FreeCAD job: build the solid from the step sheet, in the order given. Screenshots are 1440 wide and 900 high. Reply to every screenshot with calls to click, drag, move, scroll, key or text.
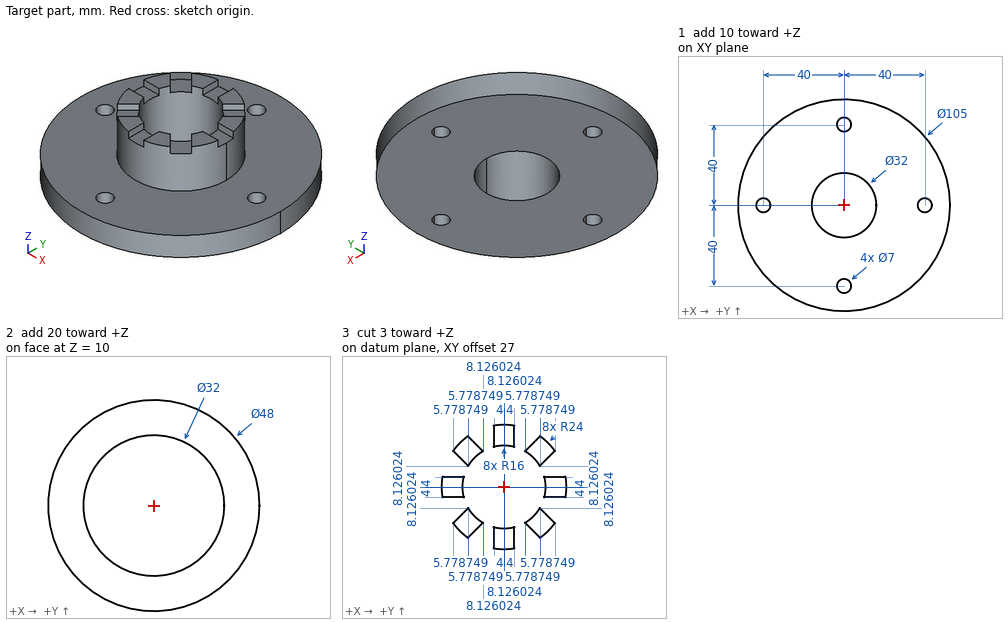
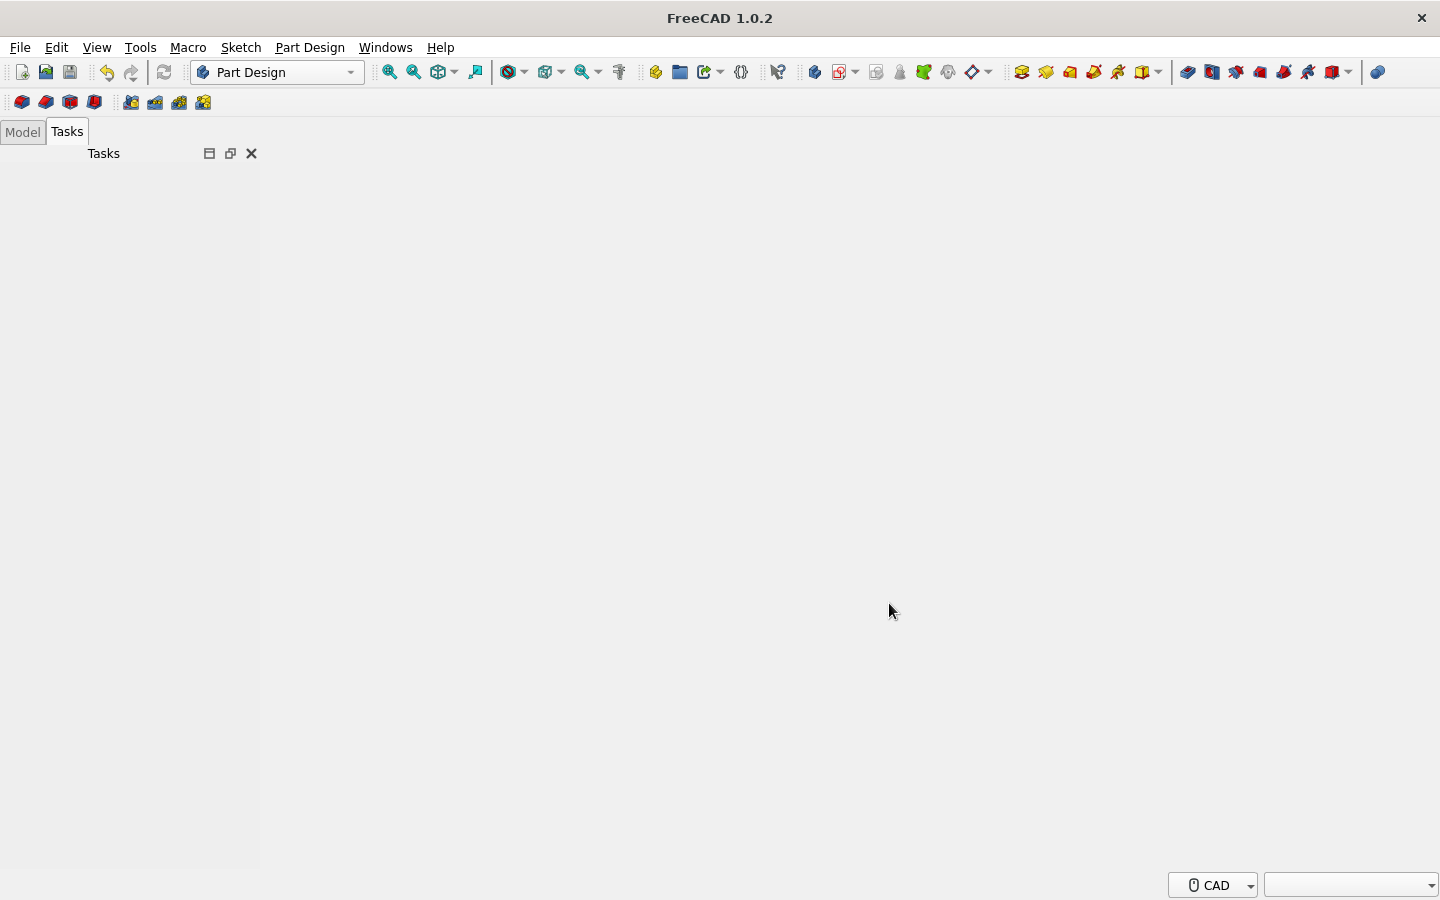
click(22, 72)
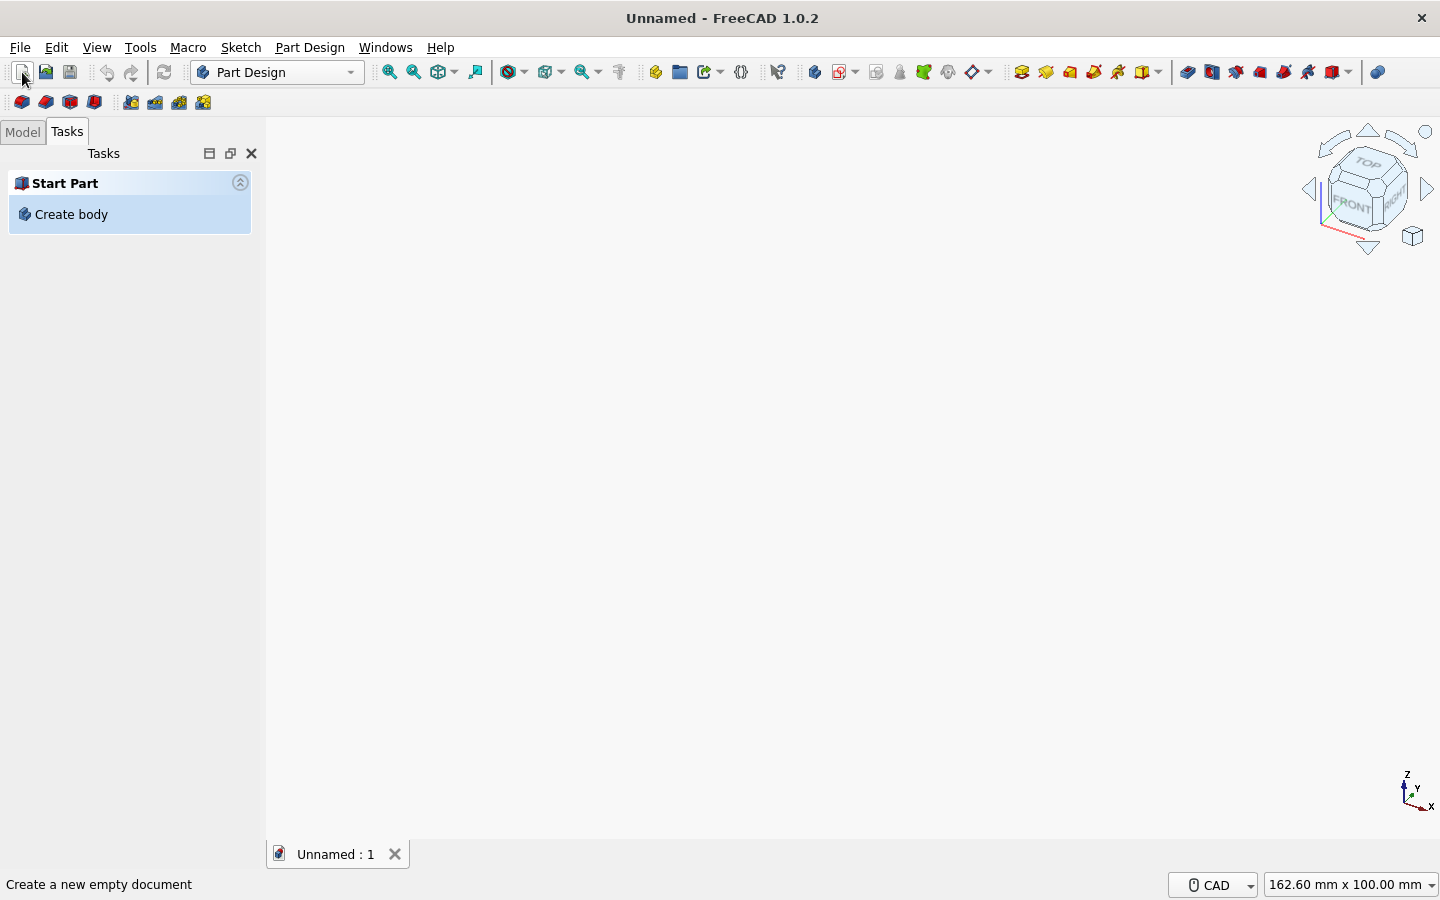
click(840, 72)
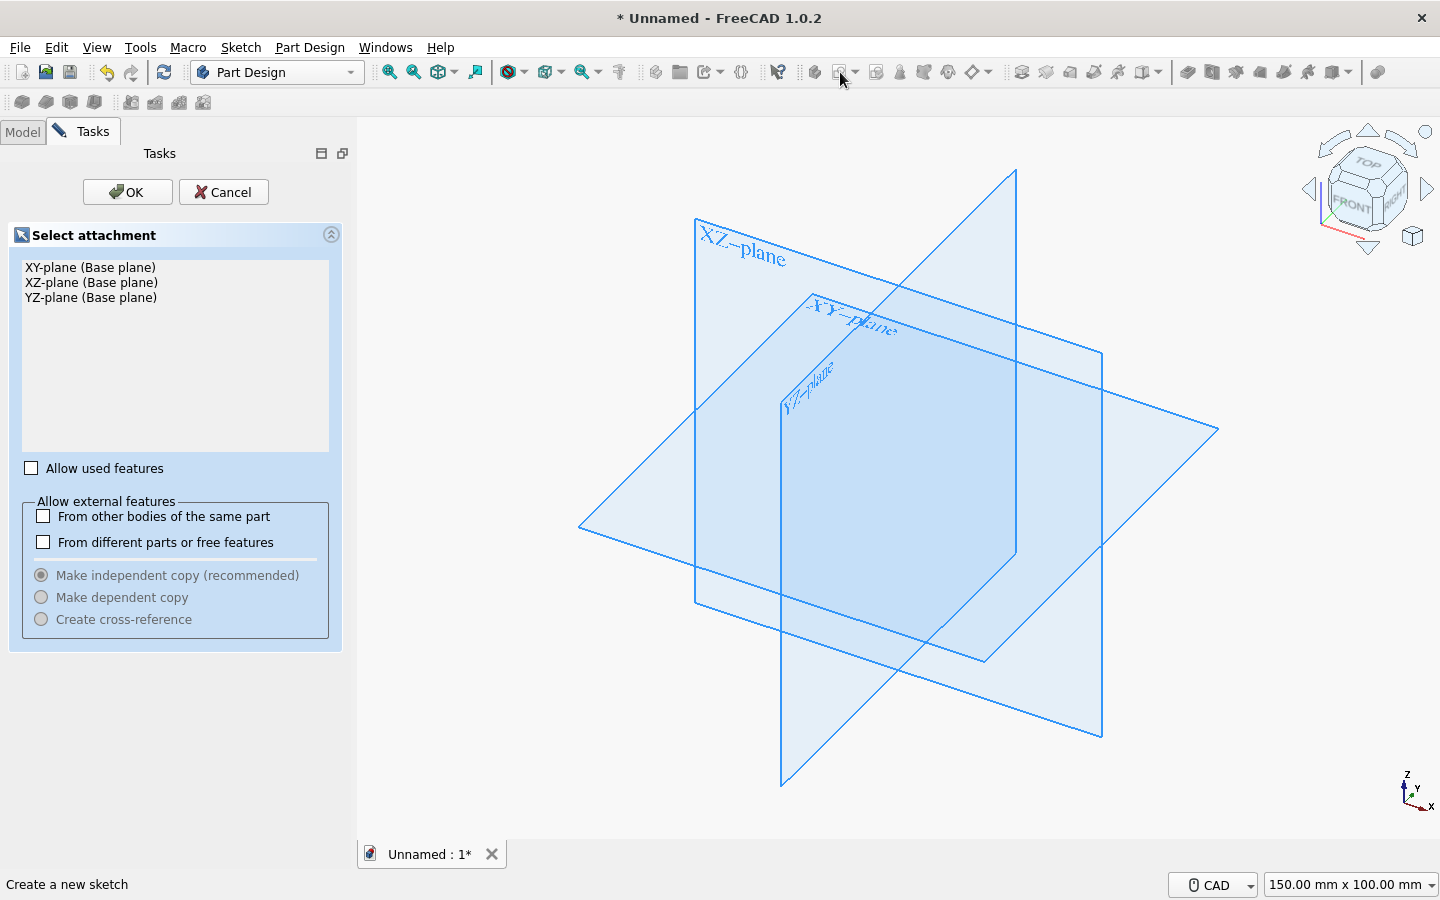
click(82, 268)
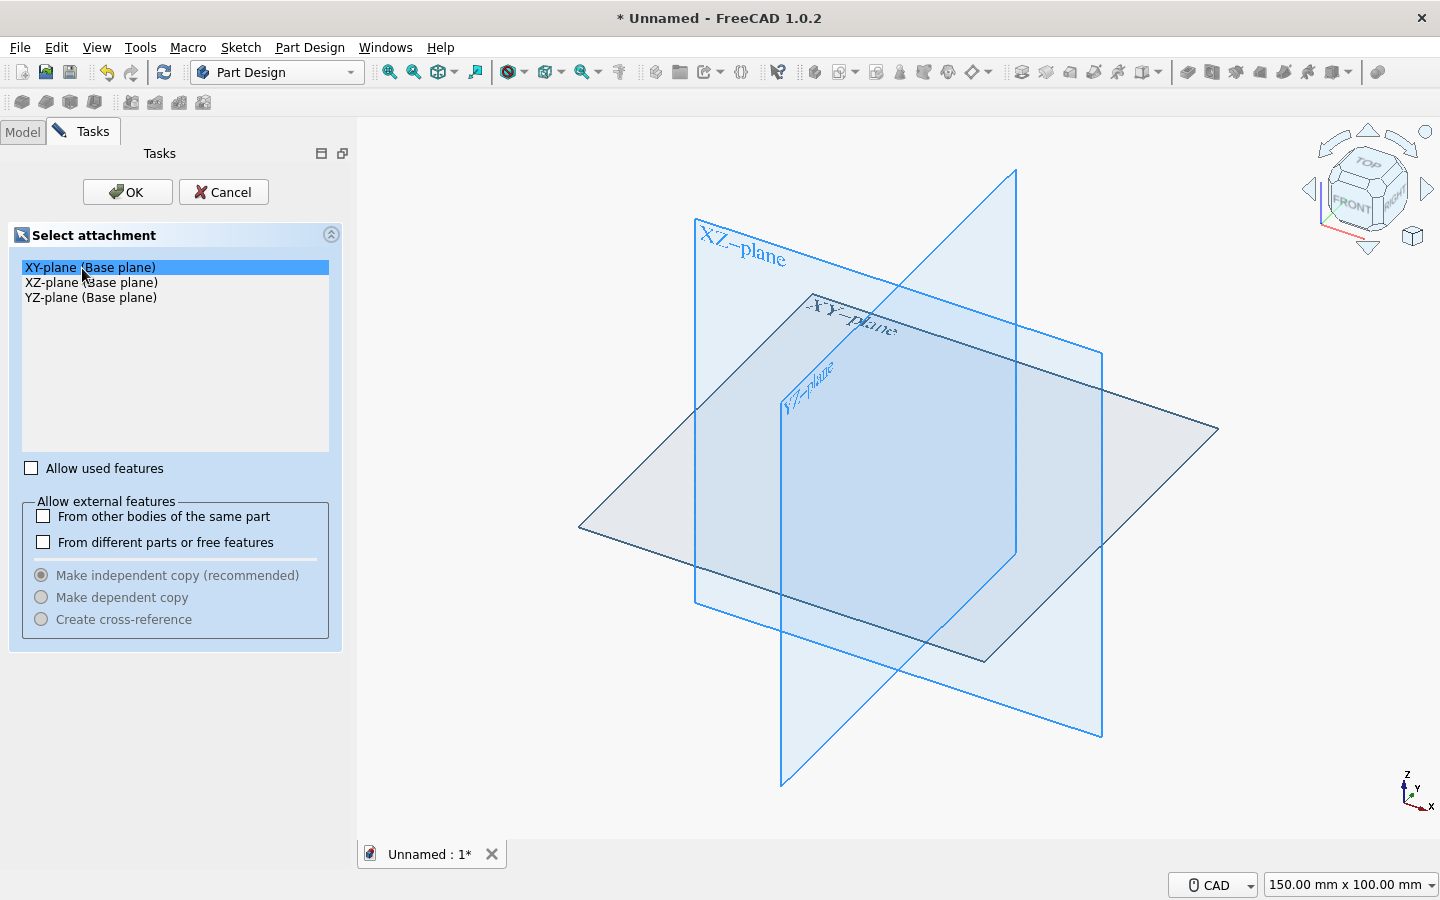
click(128, 192)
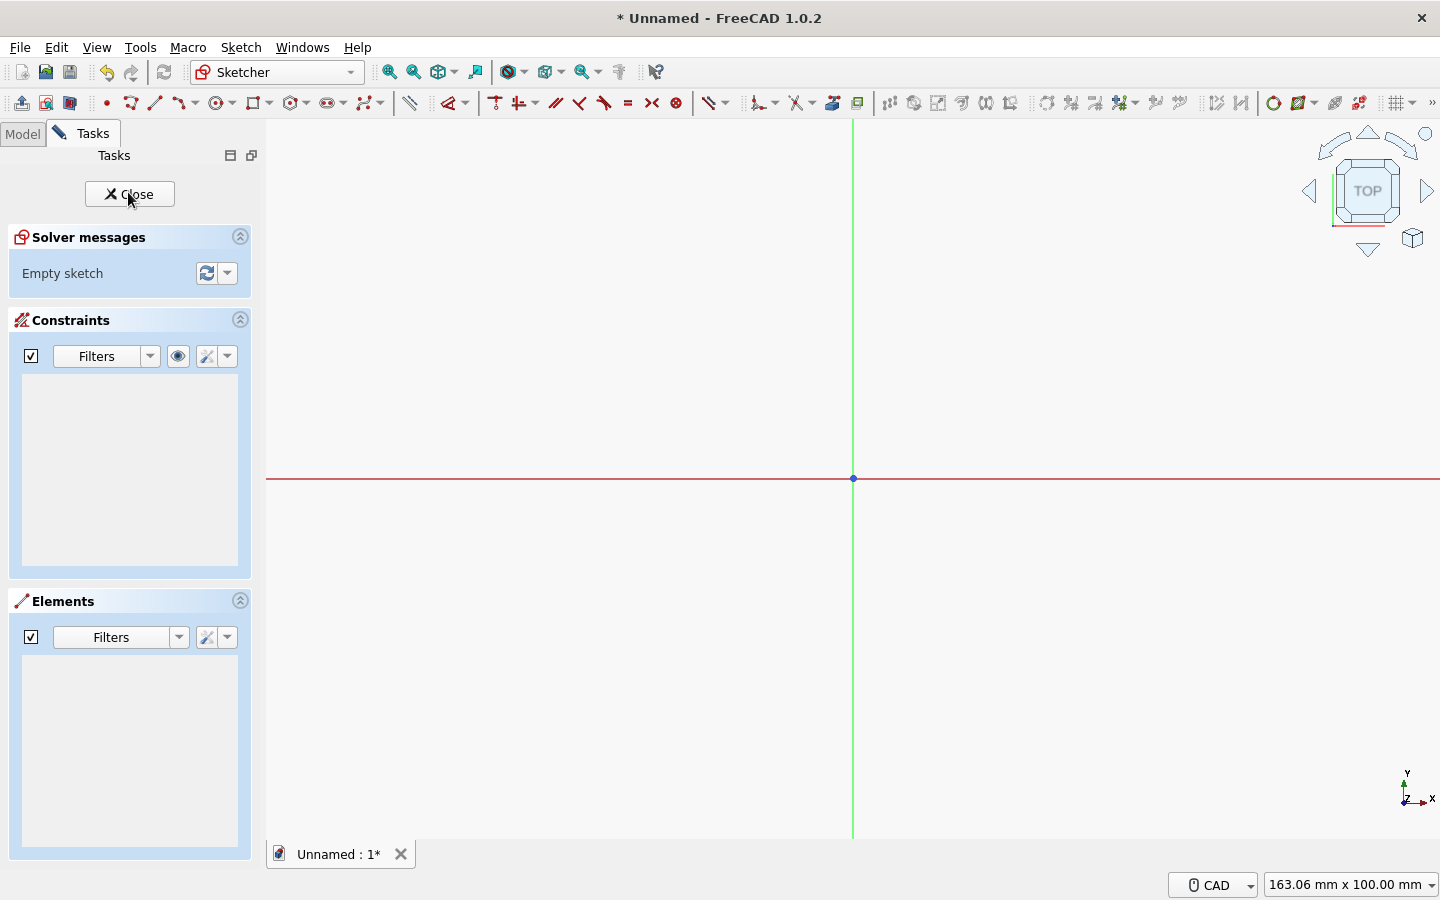
scroll(645, 479, down, 2)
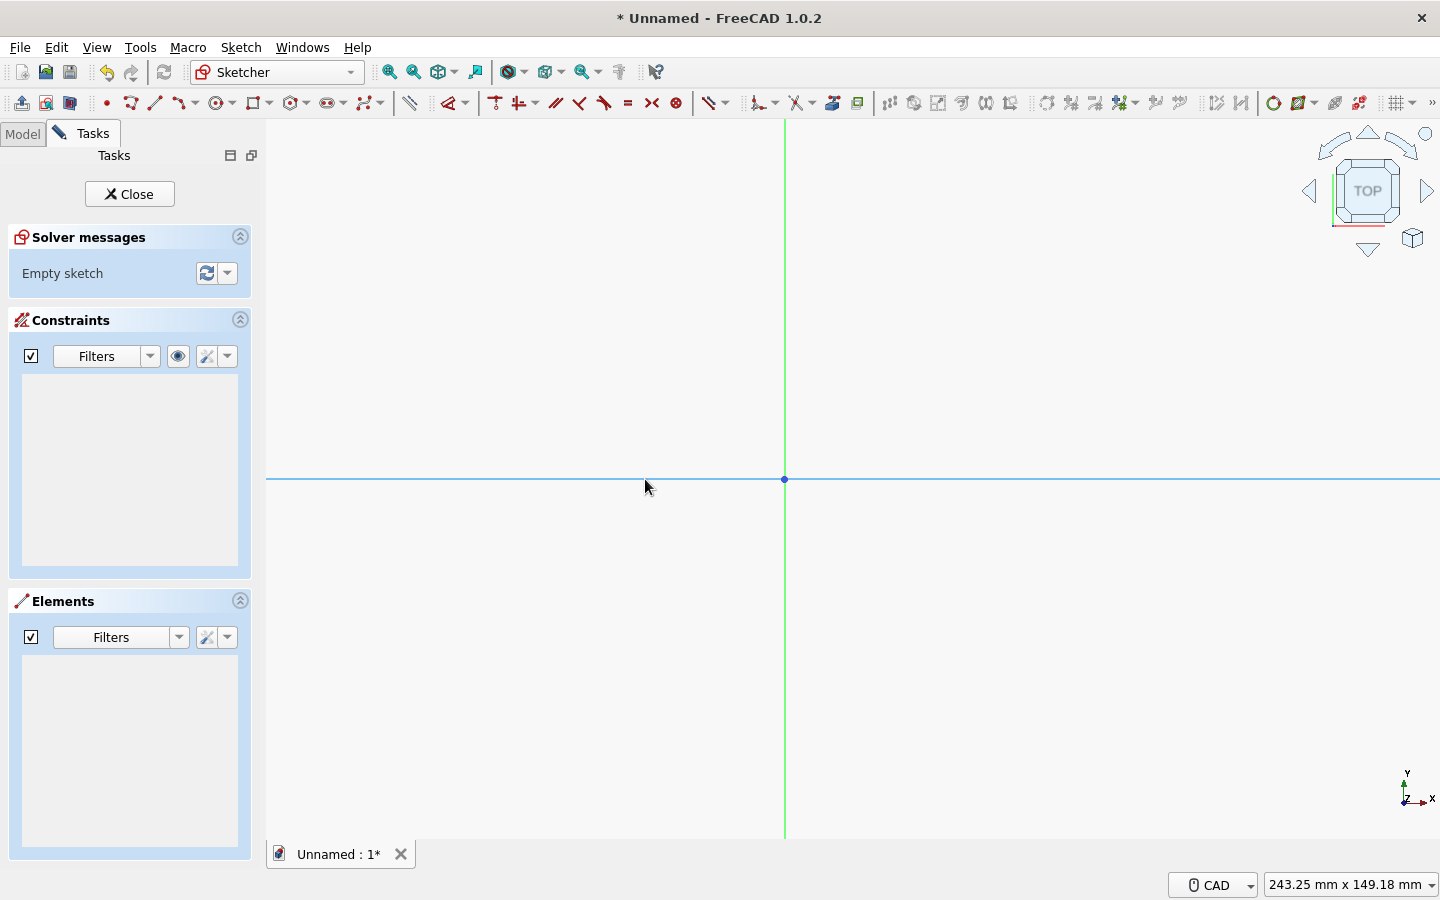
click(216, 104)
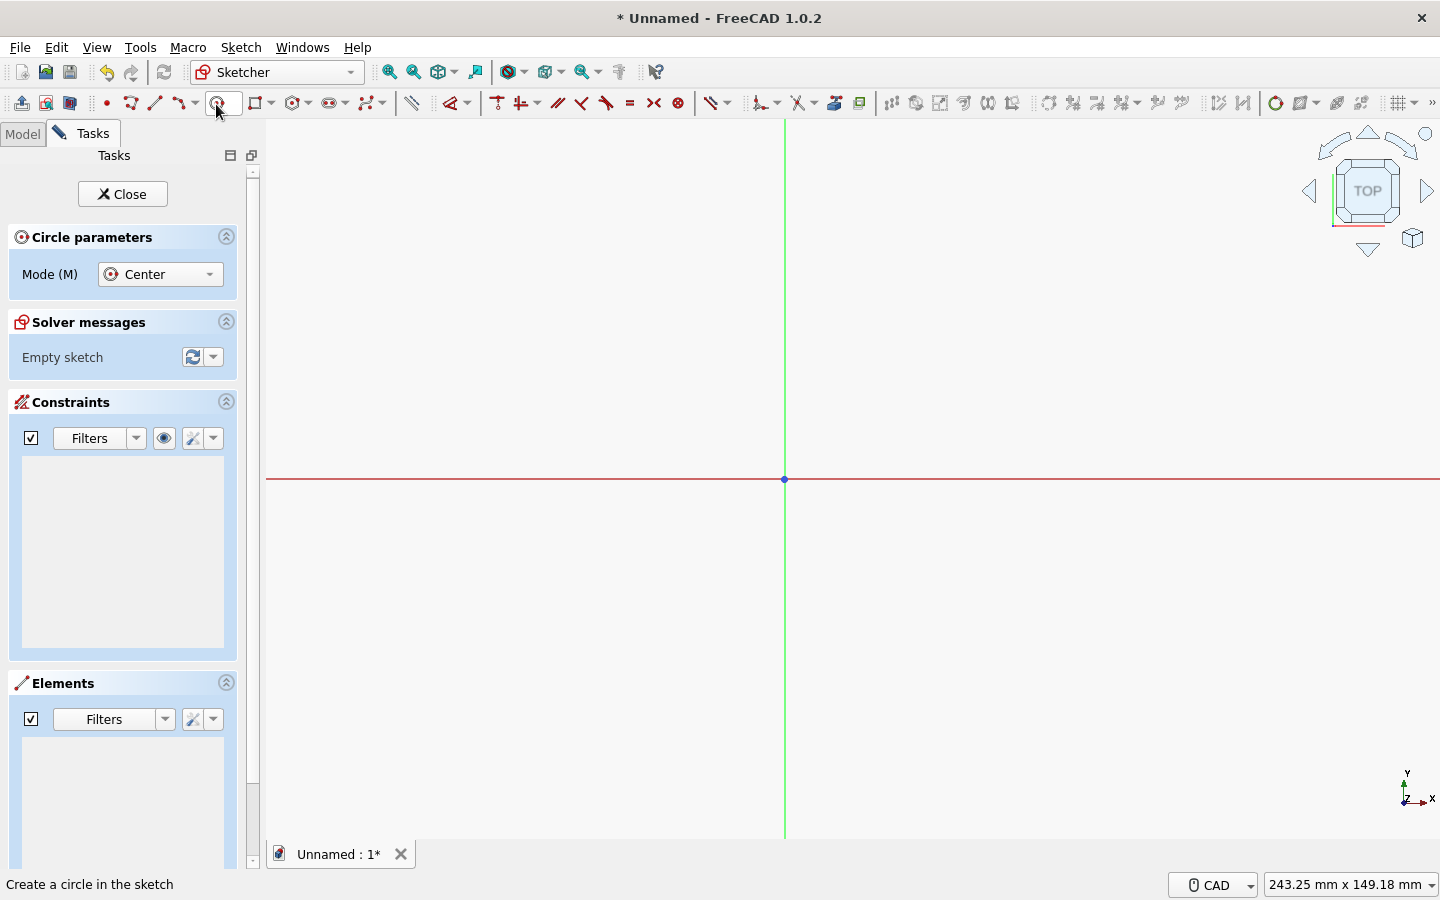
click(785, 479)
move(964, 300)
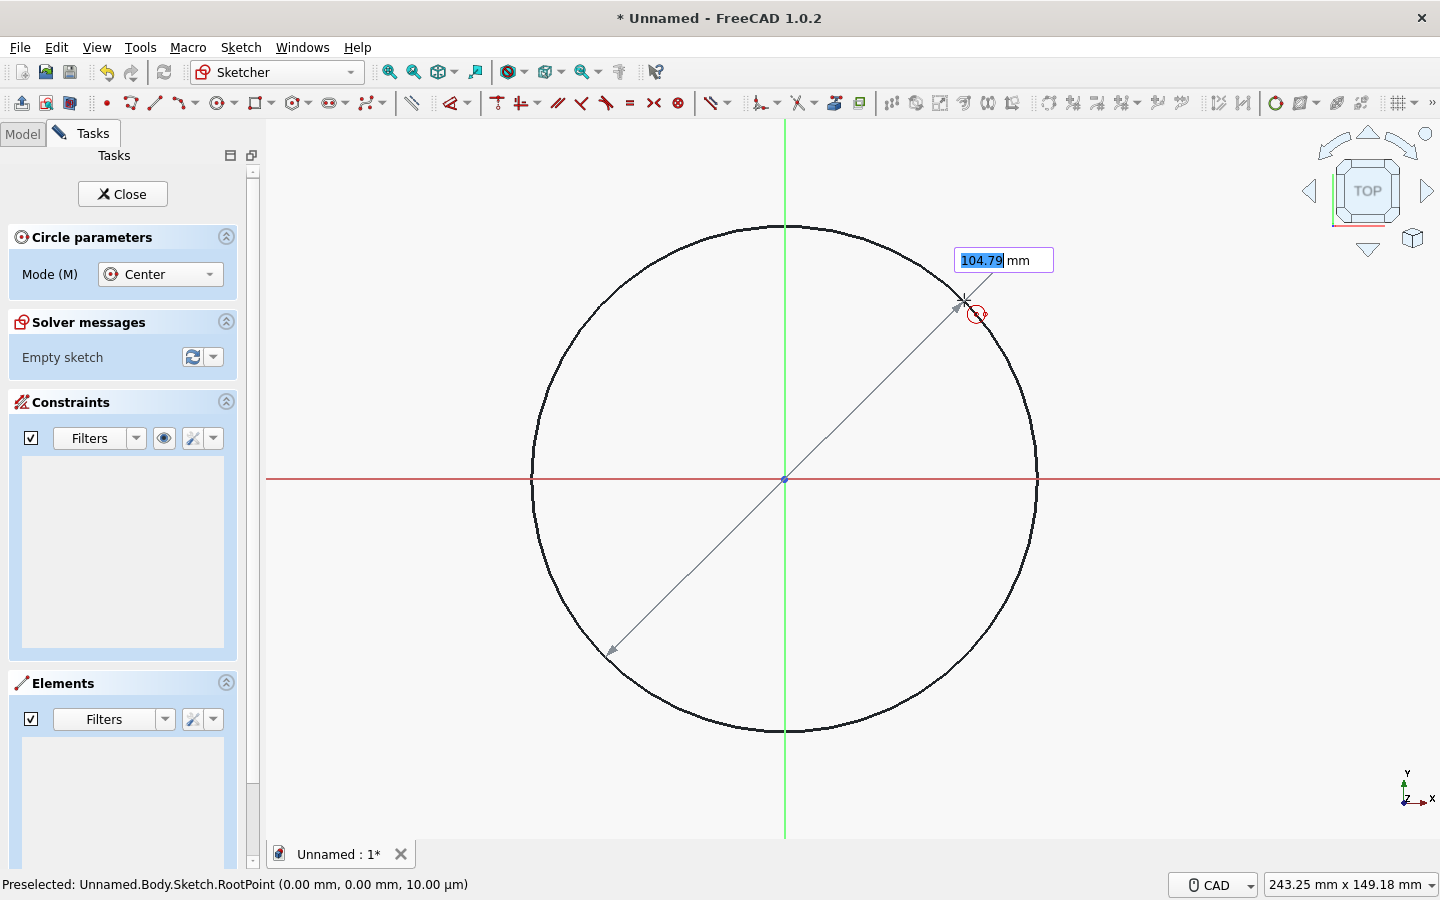
text(105)
key(Return)